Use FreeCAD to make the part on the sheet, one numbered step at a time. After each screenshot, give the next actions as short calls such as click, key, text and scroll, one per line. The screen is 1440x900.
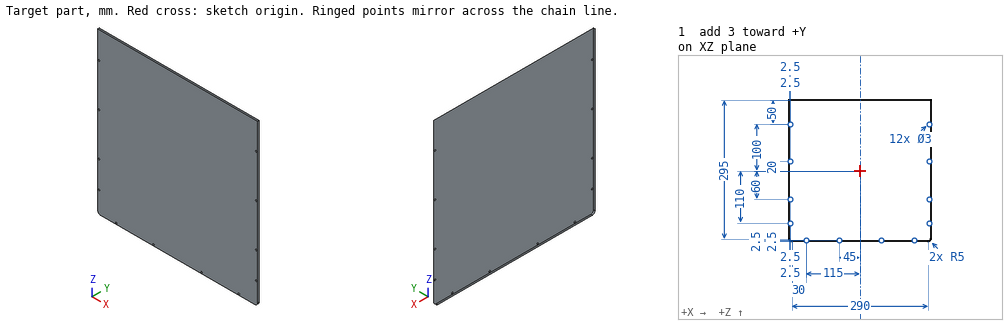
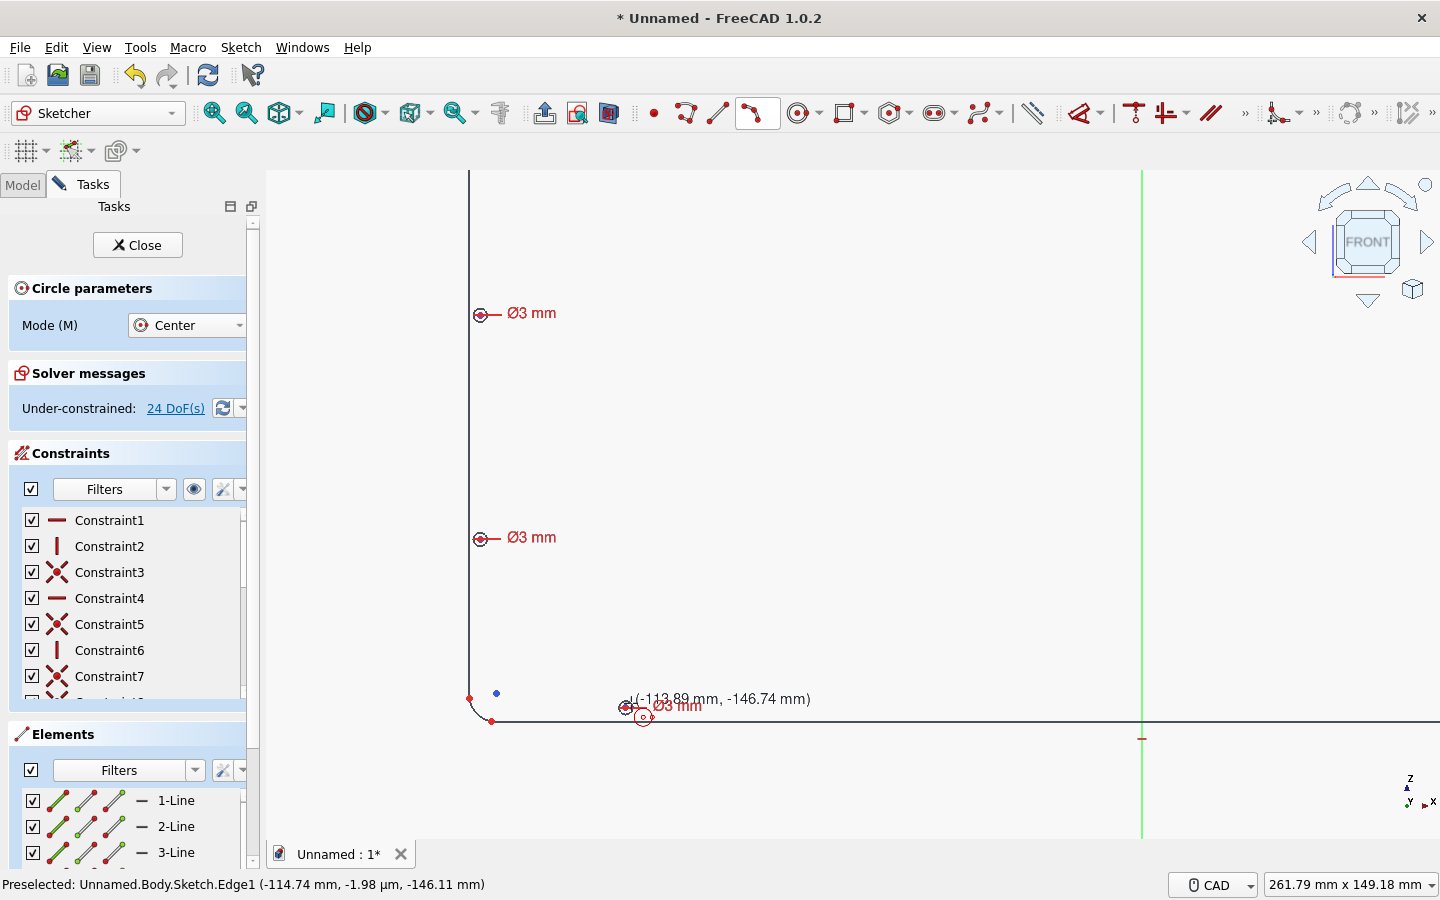
scroll(940, 707, up, 7)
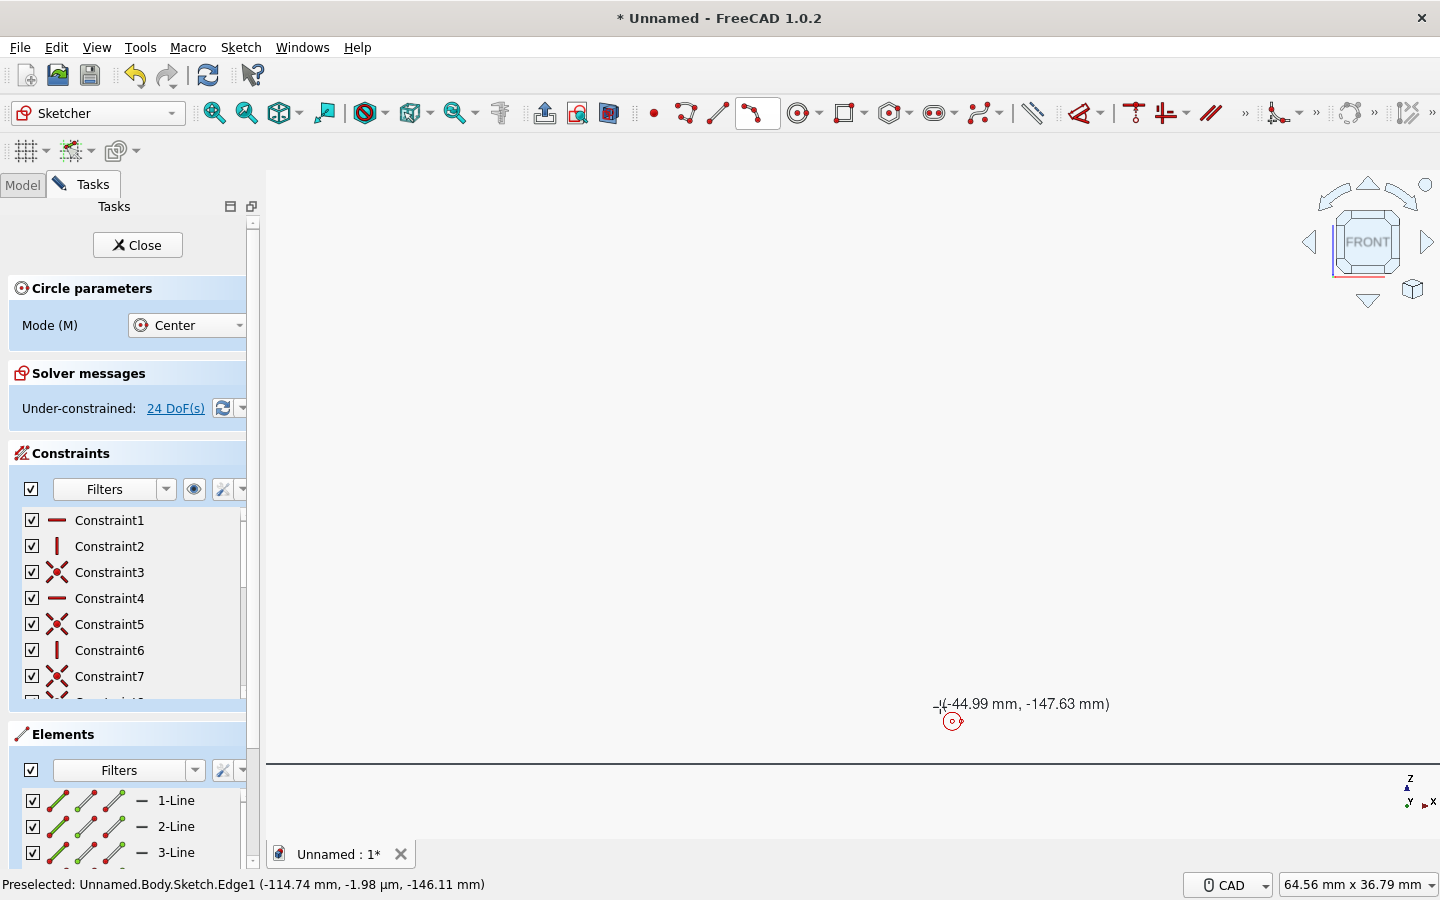
click(938, 706)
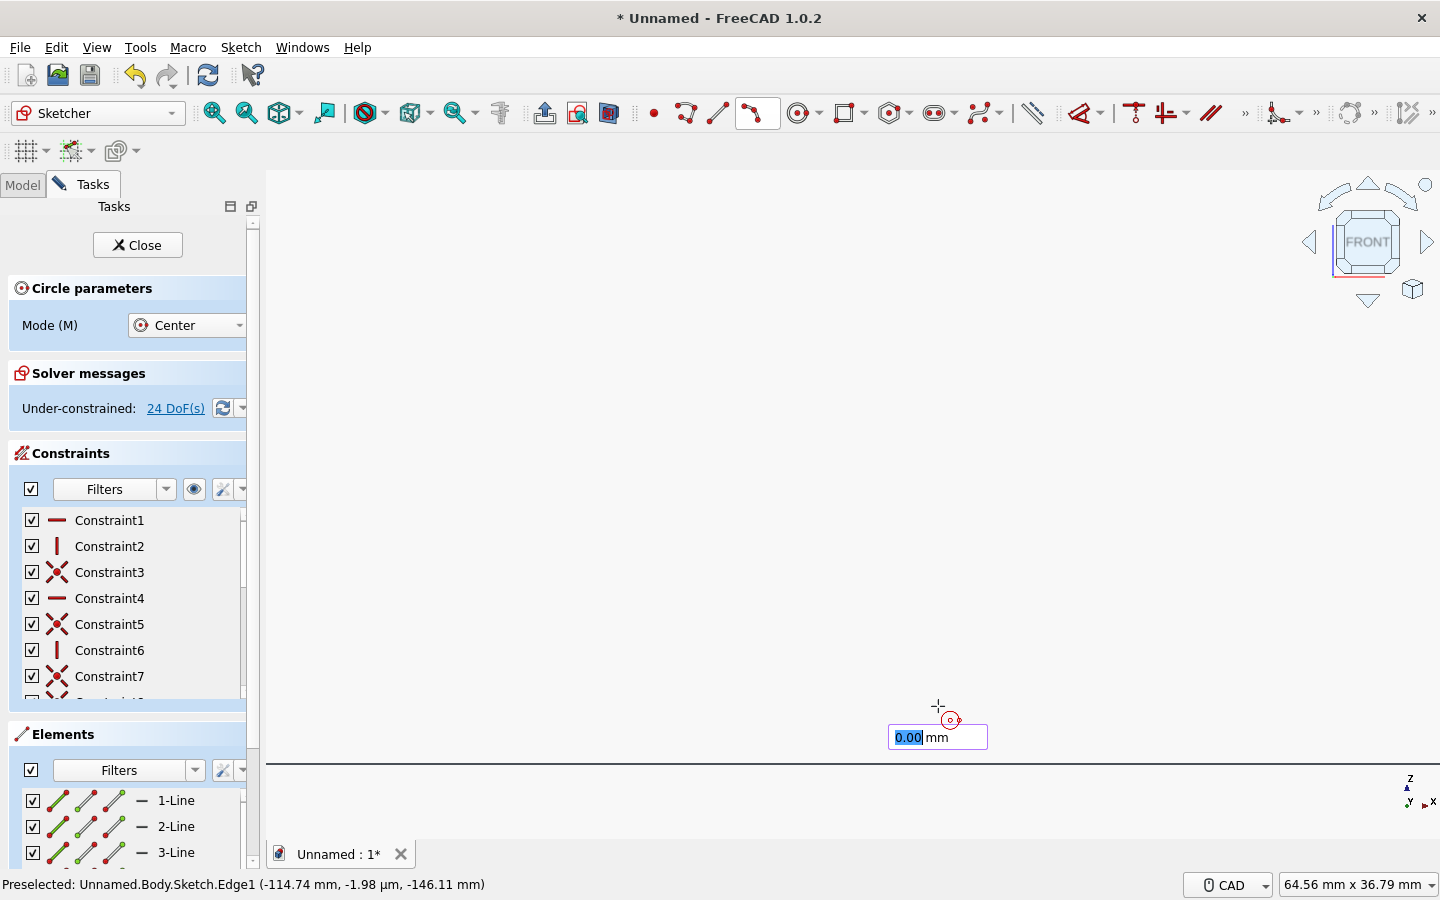
scroll(707, 704, down, 13)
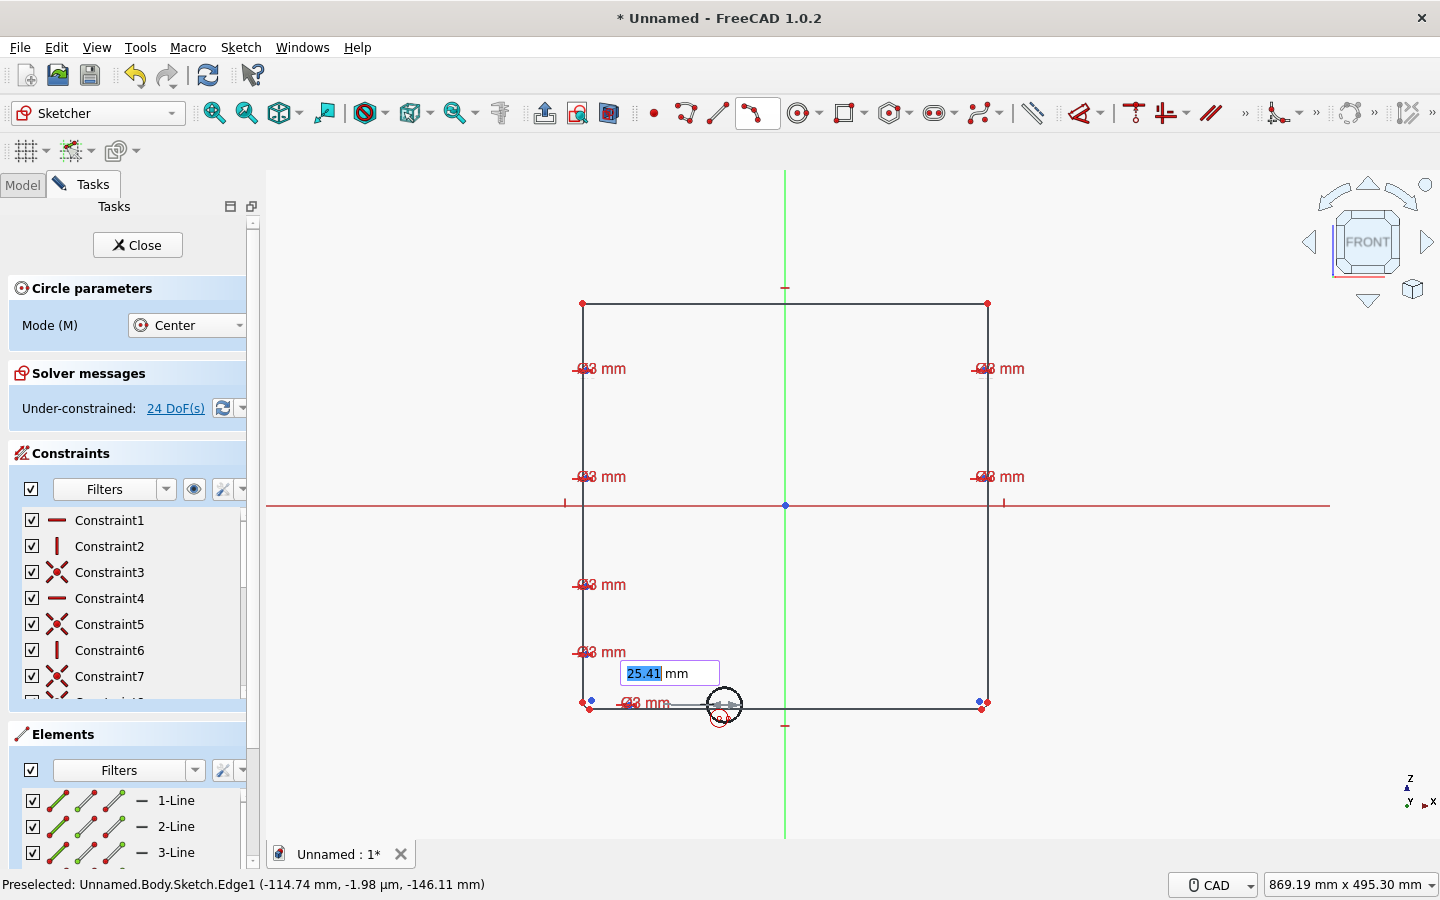
scroll(726, 703, up, 6)
move(725, 703)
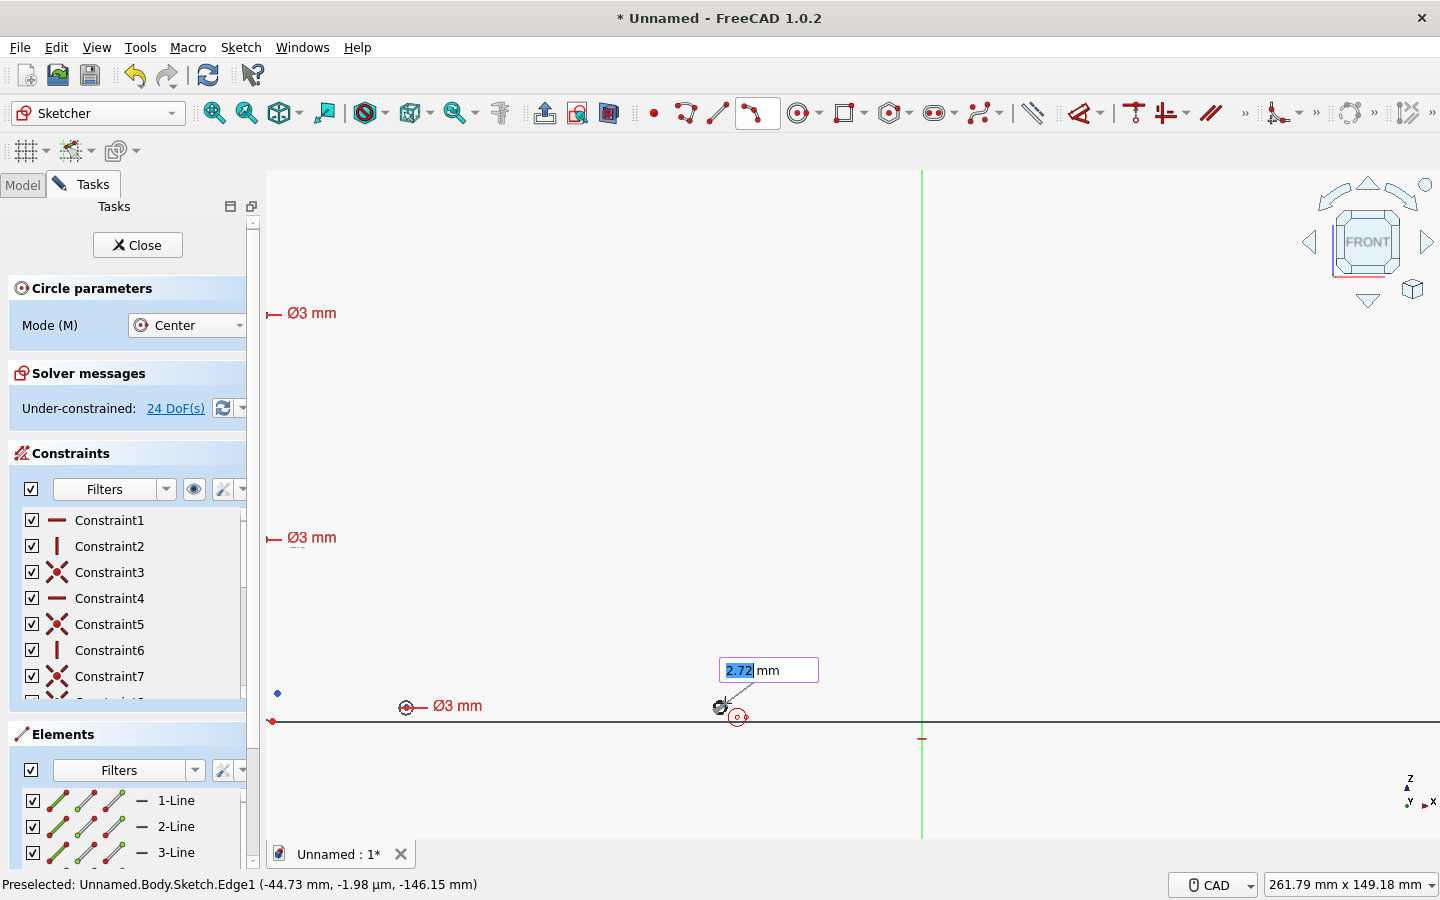
text(3)
key(Return)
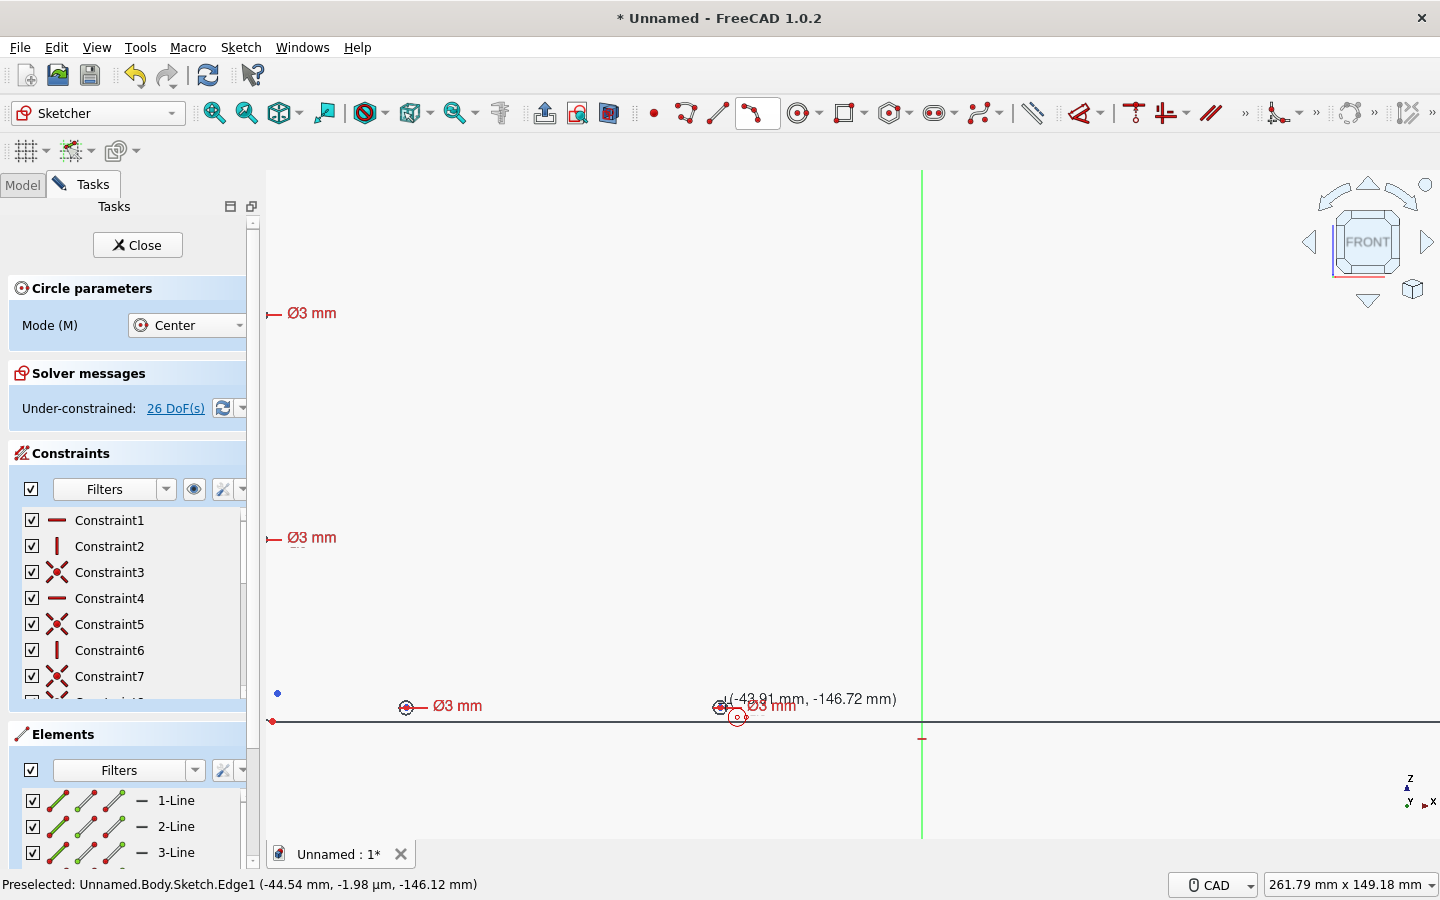
scroll(725, 702, down, 6)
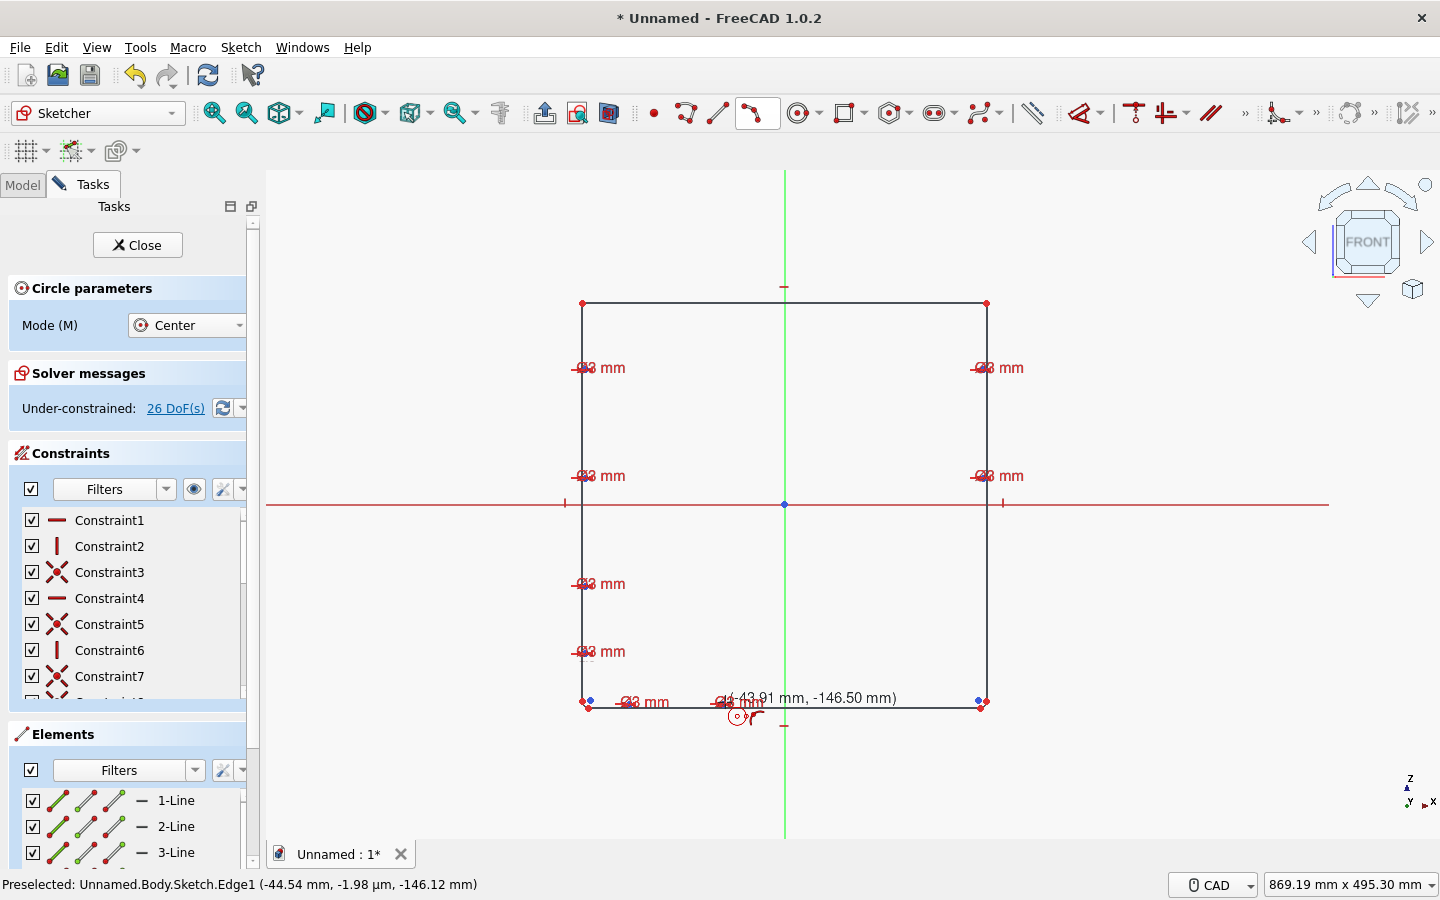
scroll(984, 586, up, 13)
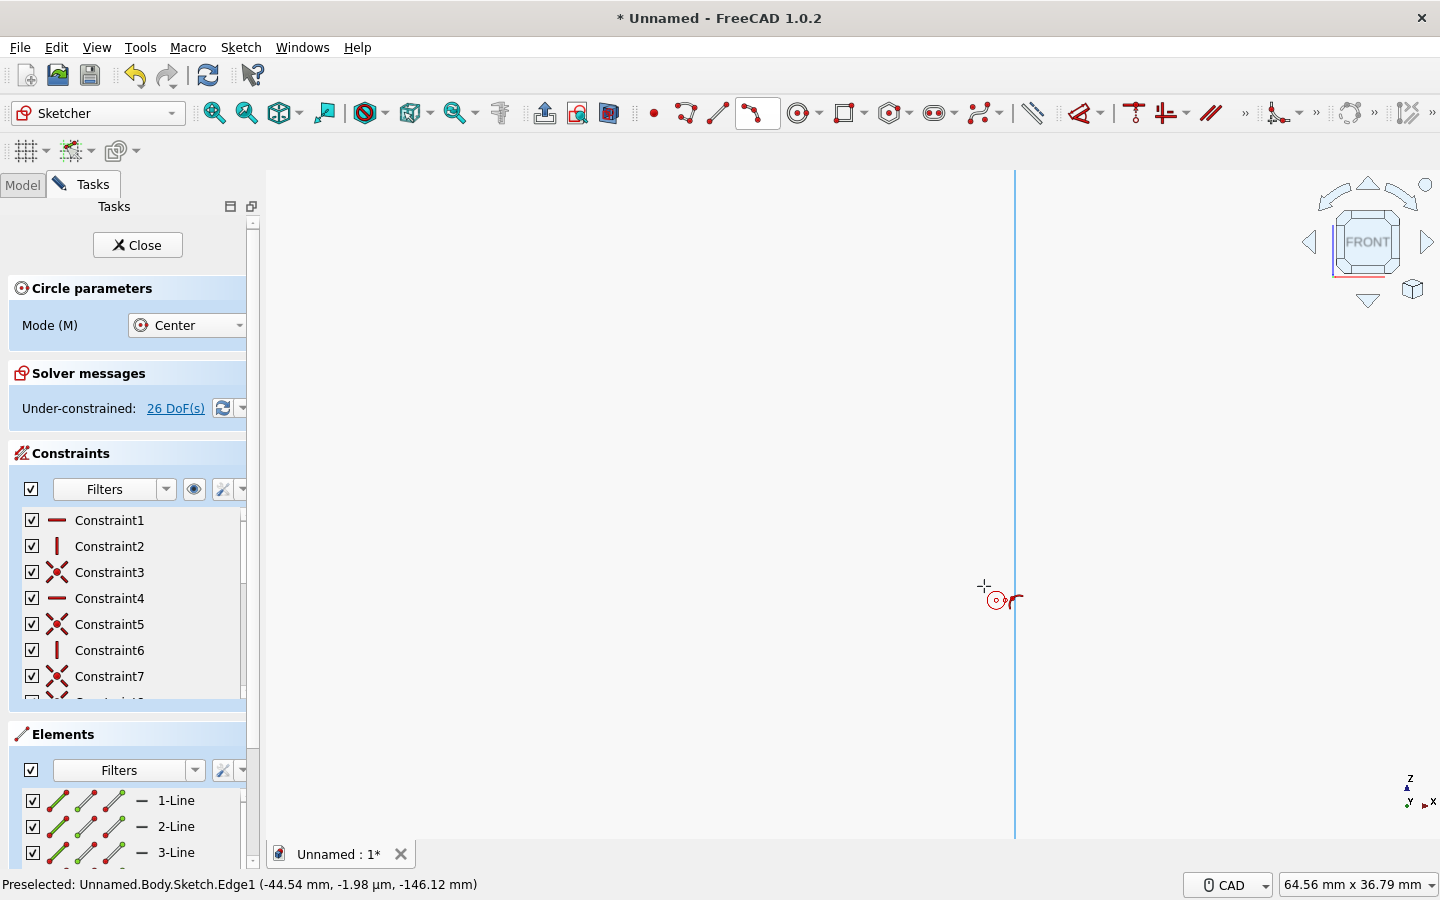
click(974, 579)
move(993, 559)